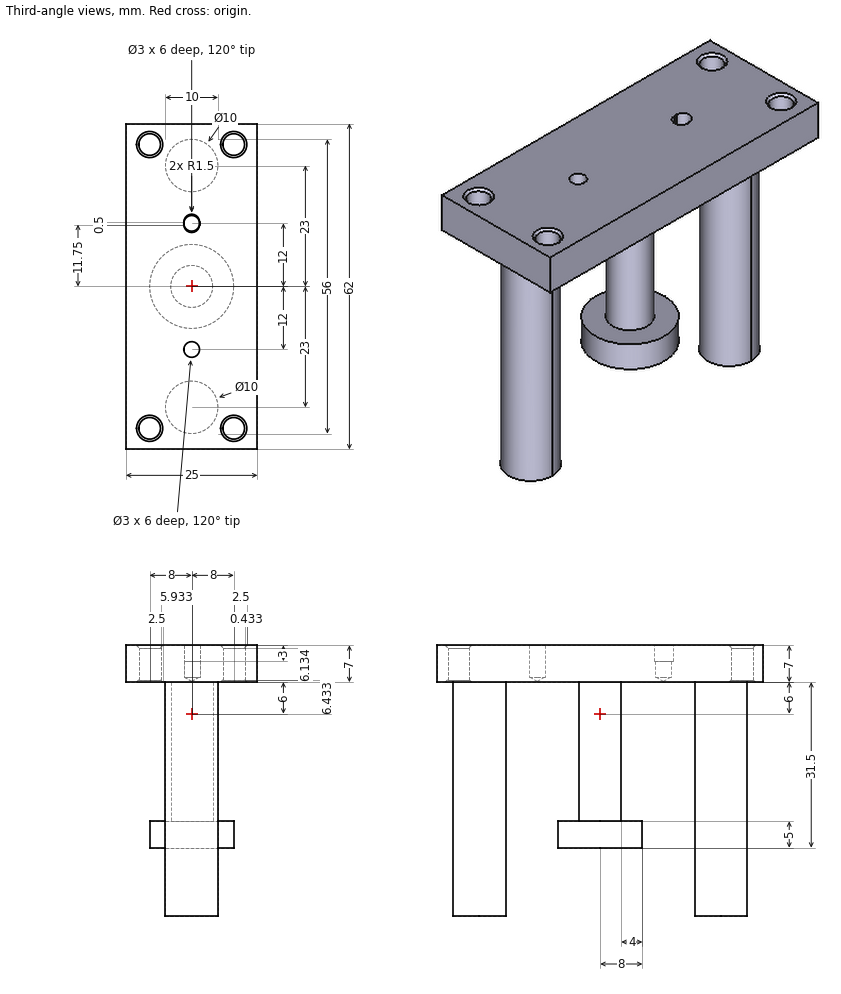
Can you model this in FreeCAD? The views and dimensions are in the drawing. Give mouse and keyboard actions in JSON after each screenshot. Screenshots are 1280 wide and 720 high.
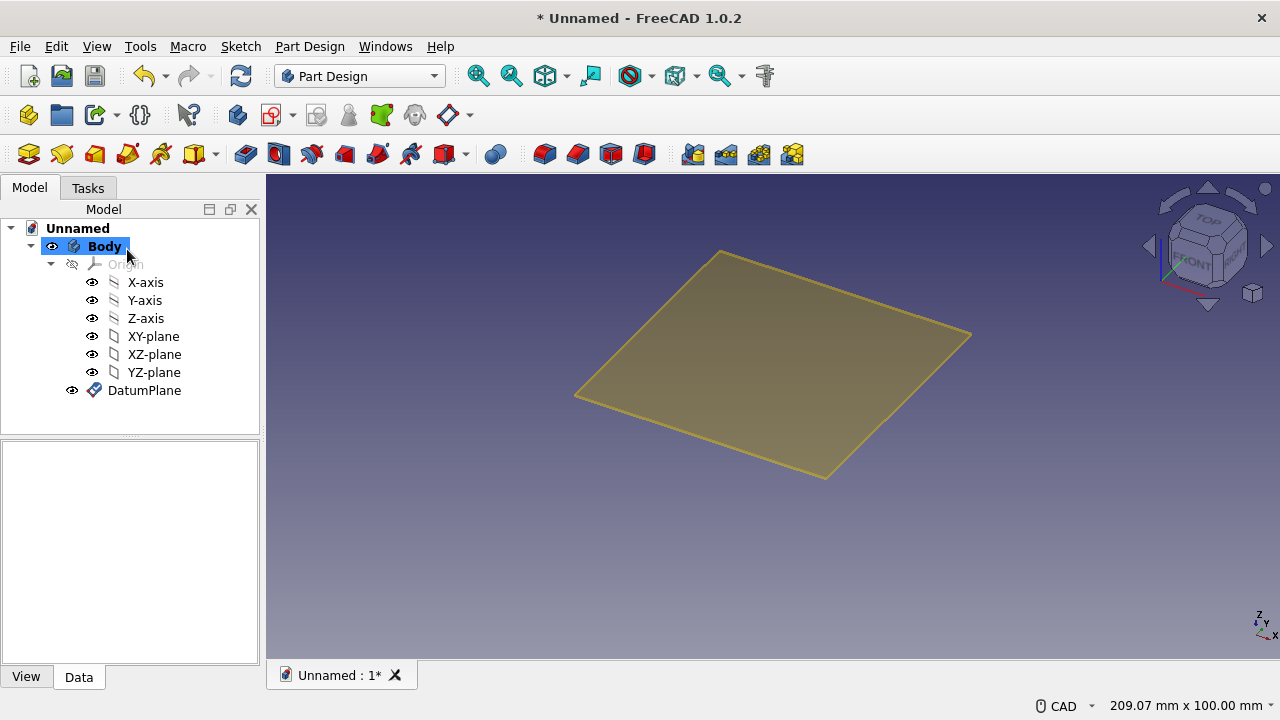
{"action": "left_click", "coordinate": [117, 390]}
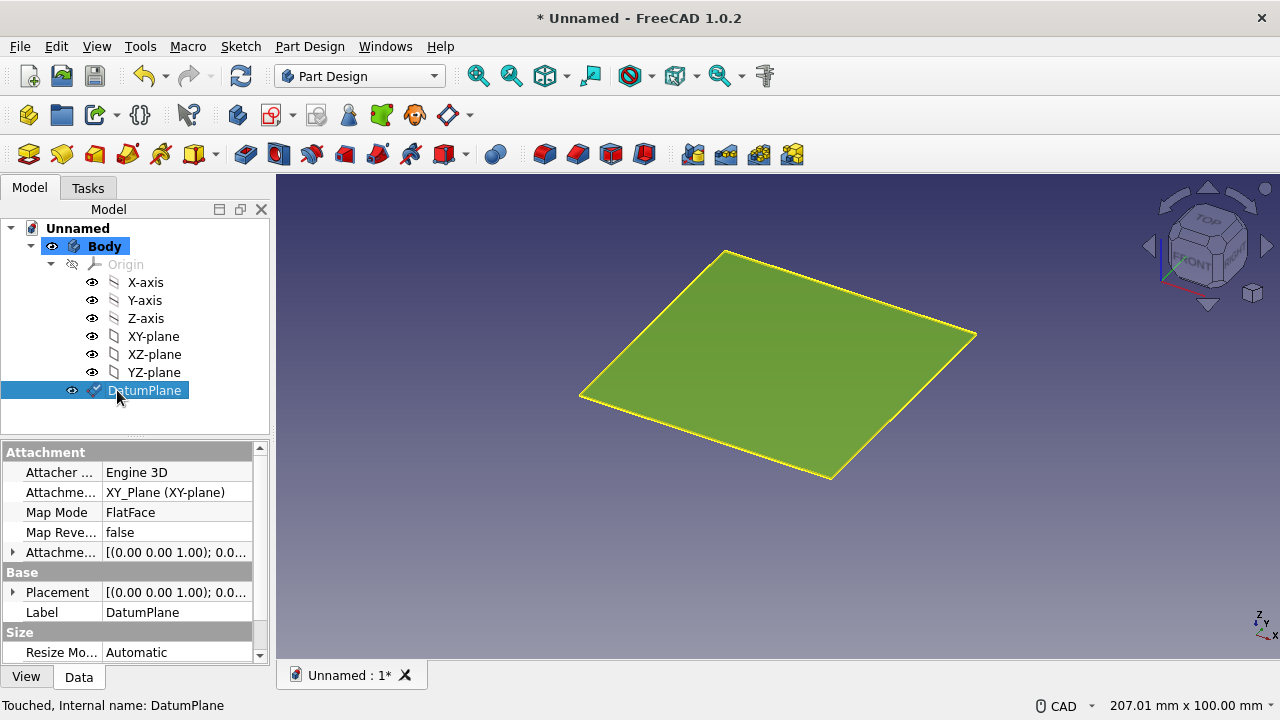
{"action": "left_click", "coordinate": [270, 116]}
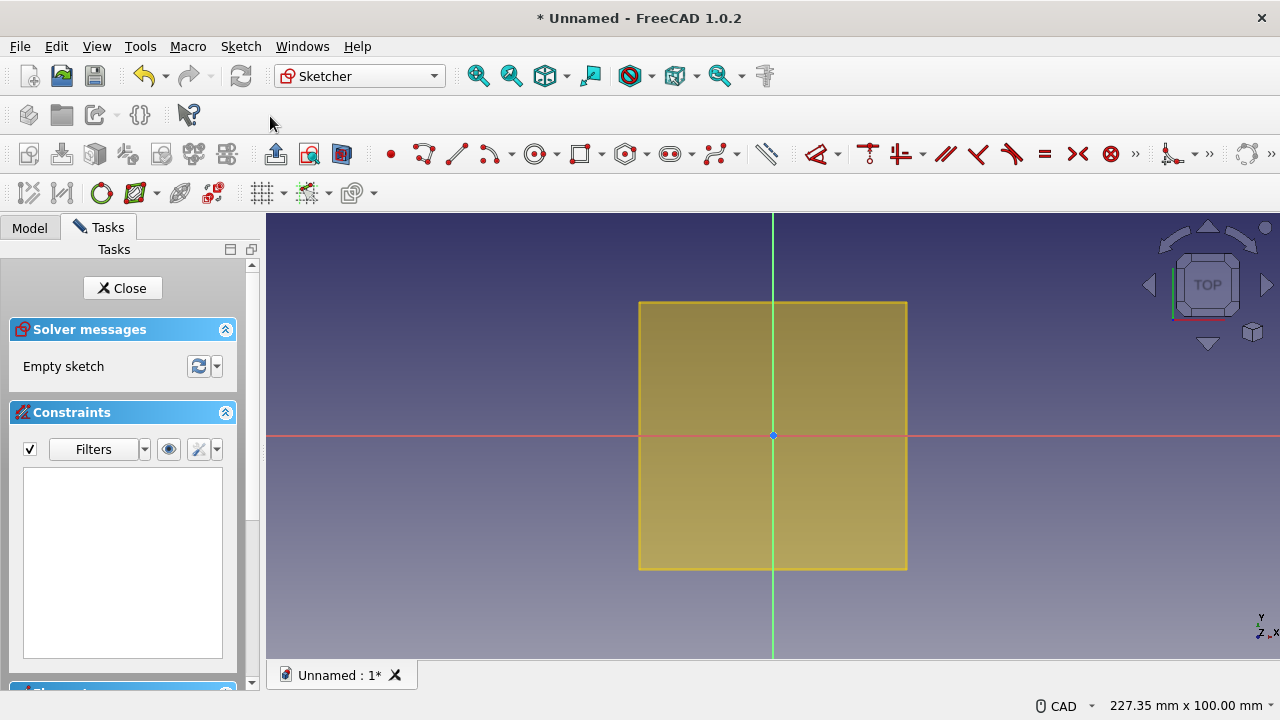
{"action": "left_click", "coordinate": [602, 154]}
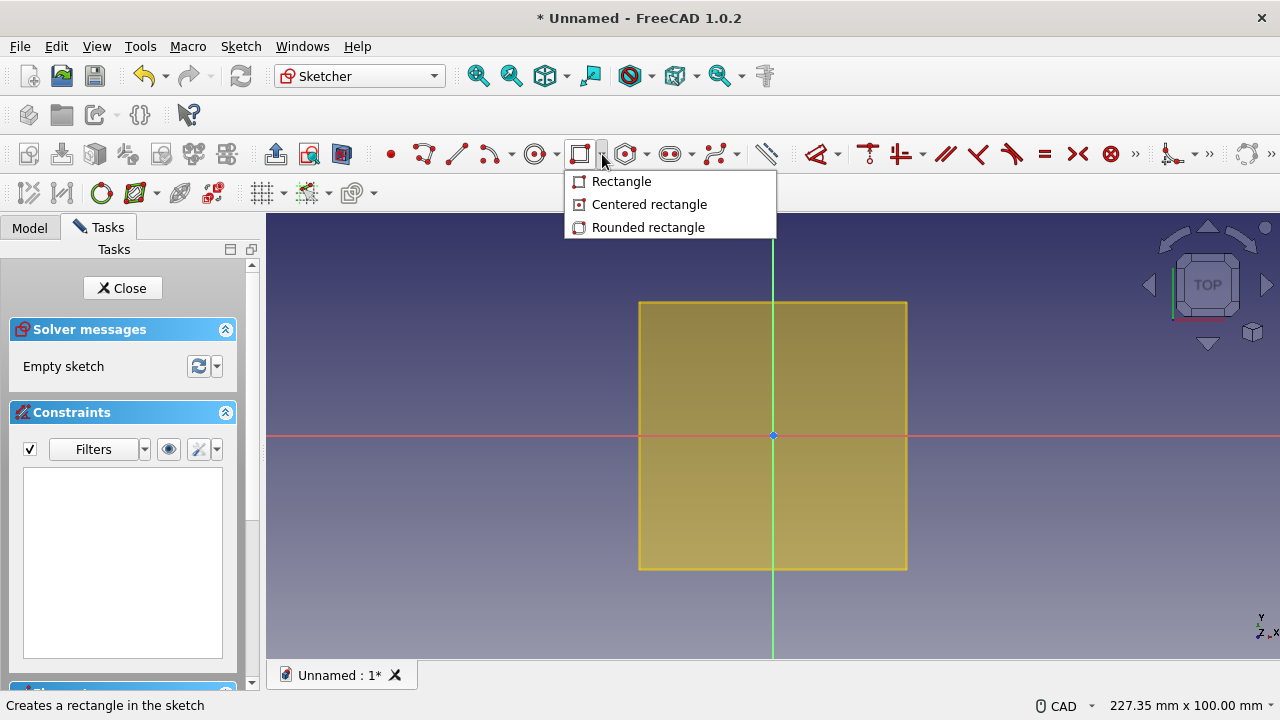
{"action": "left_click", "coordinate": [670, 204]}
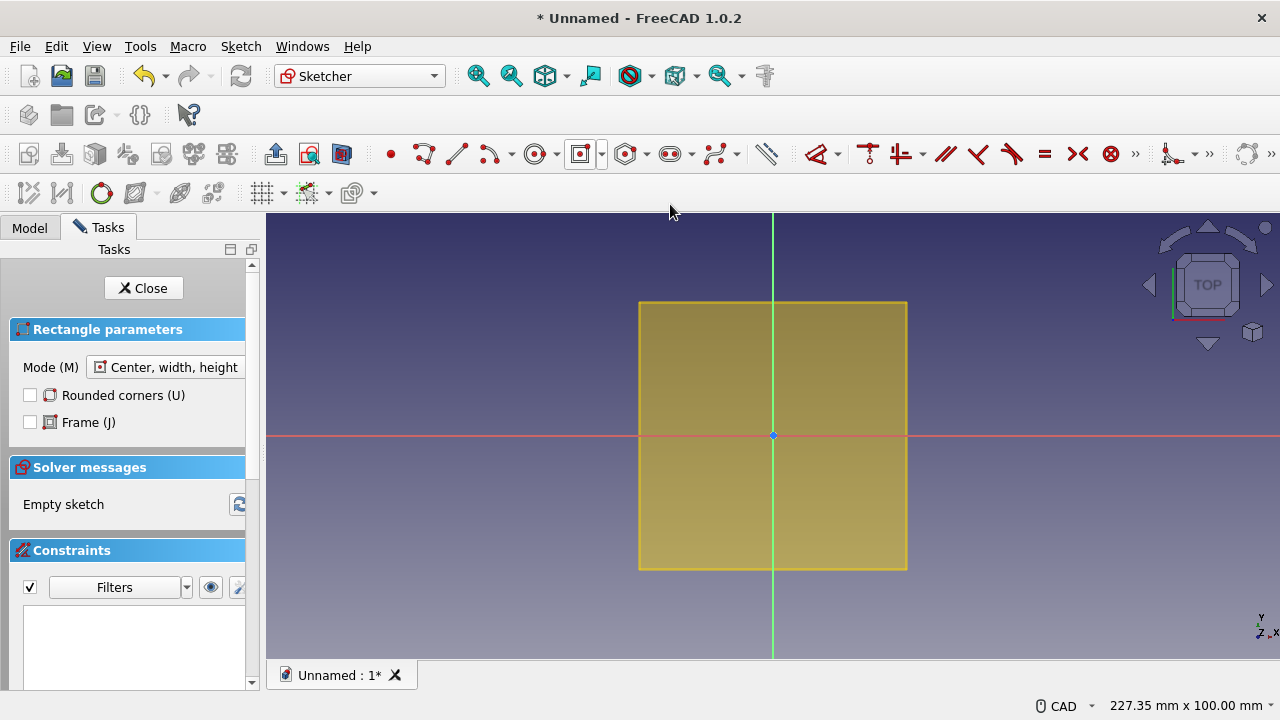
{"action": "left_click", "coordinate": [773, 436]}
{"action": "left_click", "coordinate": [829, 298]}
{"action": "key", "text": "Escape"}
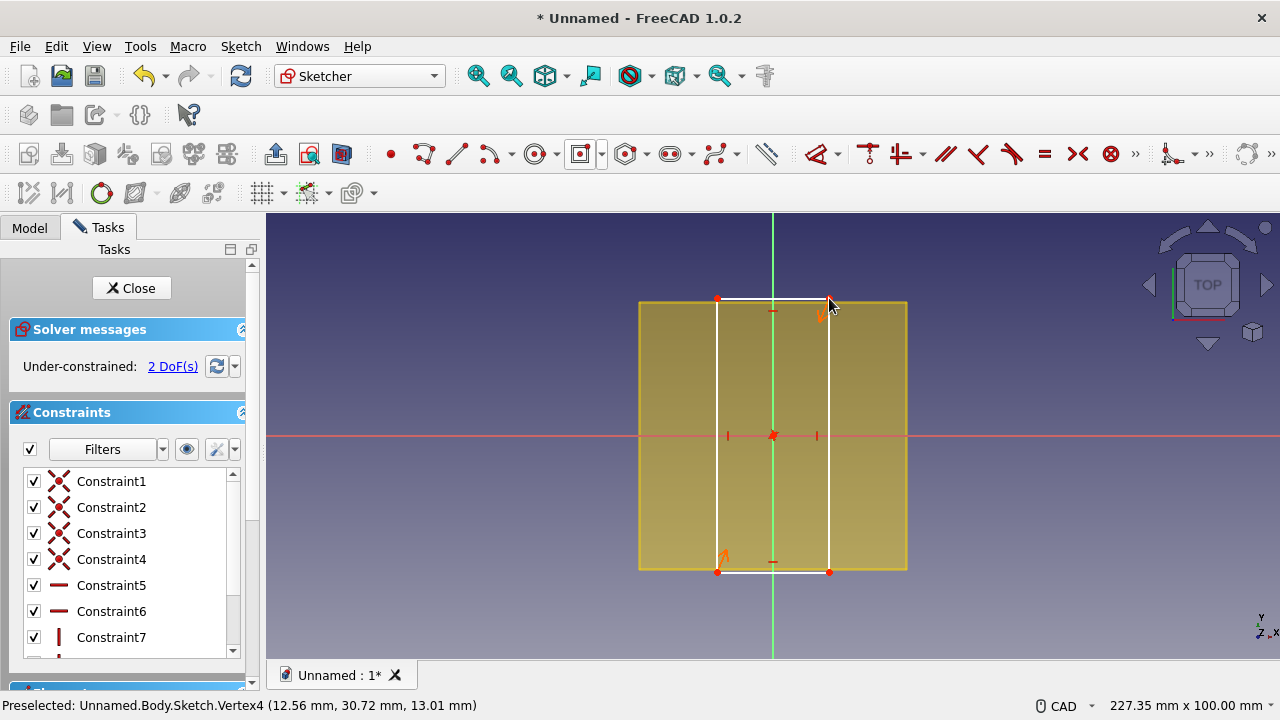
{"action": "left_click", "coordinate": [816, 154]}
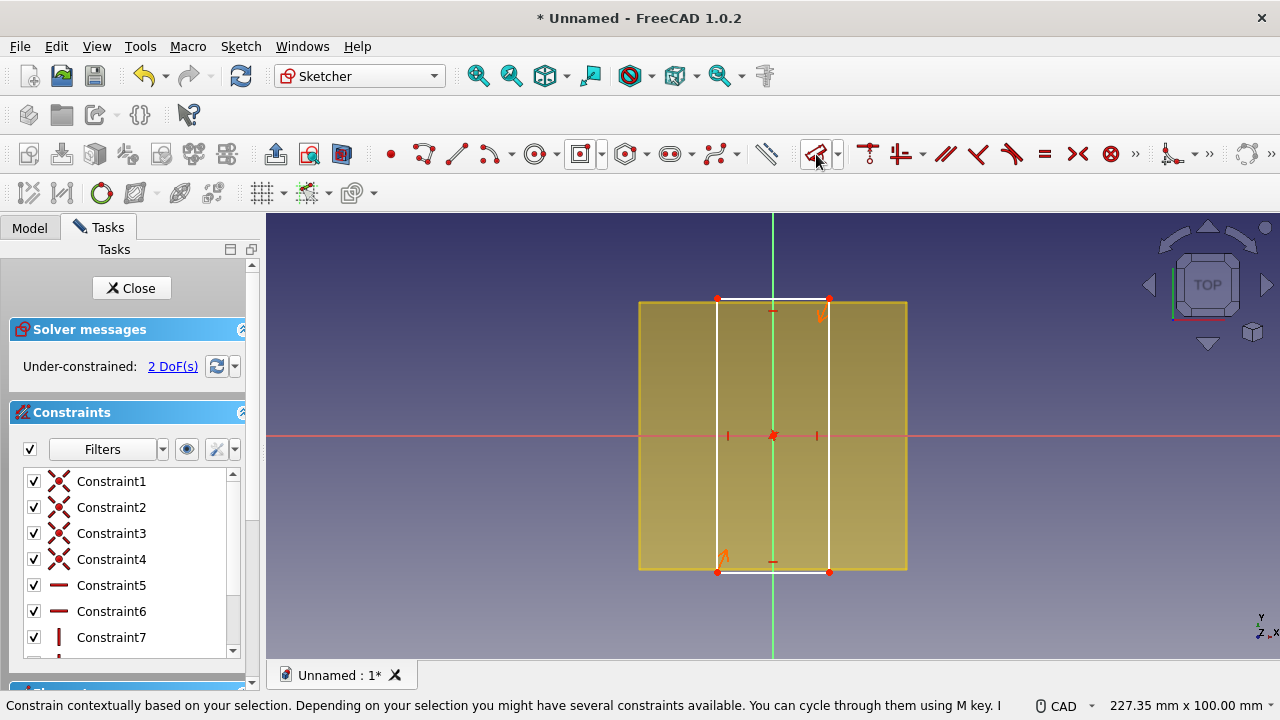
{"action": "left_click", "coordinate": [751, 573]}
{"action": "left_click", "coordinate": [747, 607]}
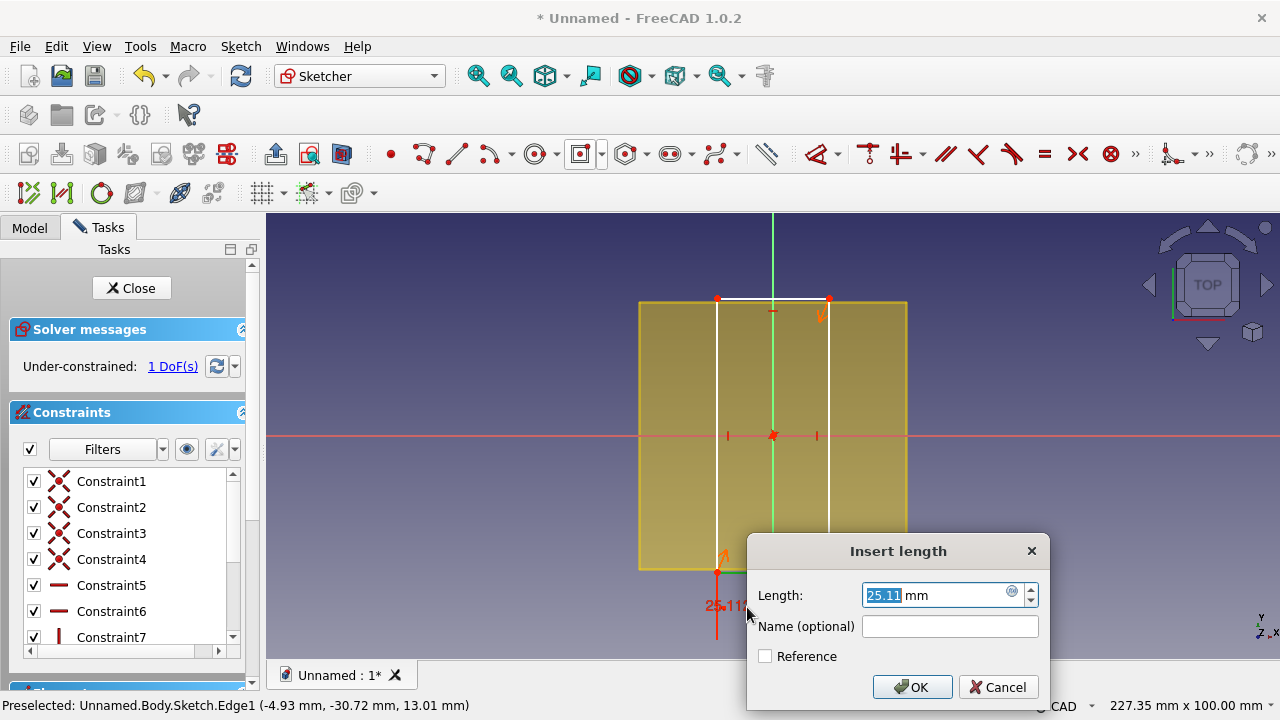
{"action": "type", "text": "25"}
{"action": "key", "text": "Return"}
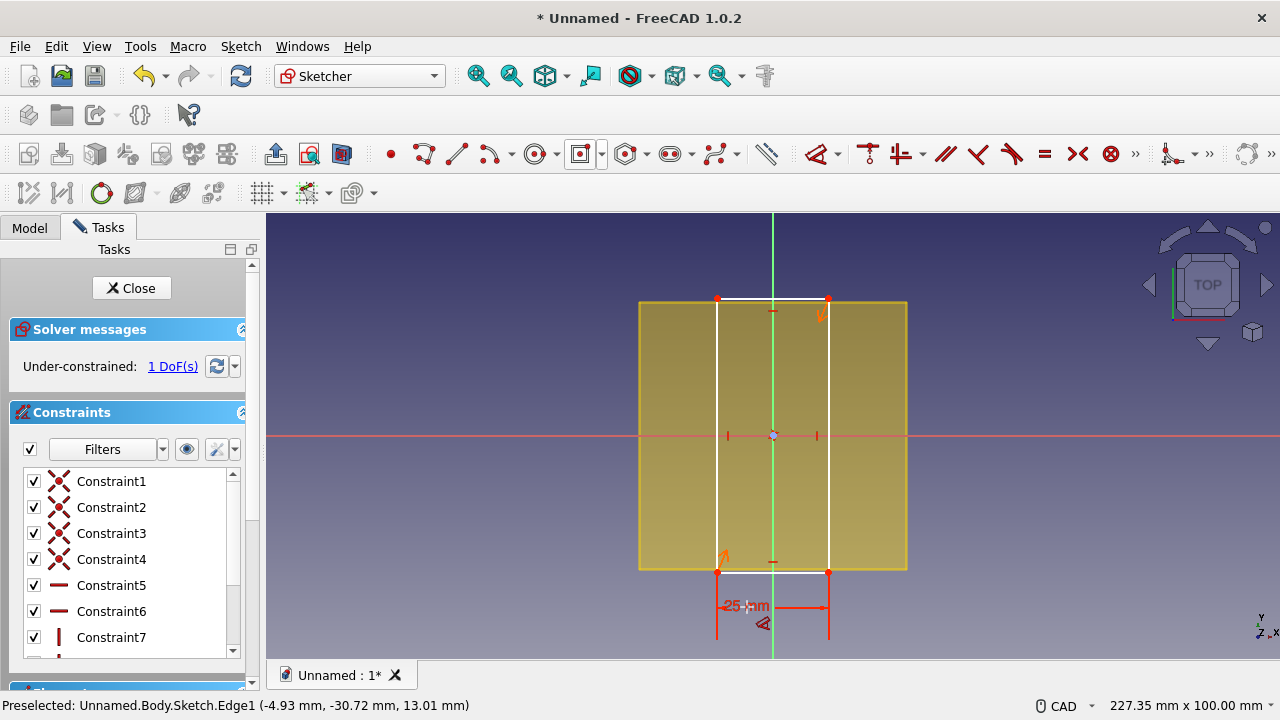
{"action": "left_click", "coordinate": [829, 491]}
{"action": "left_click", "coordinate": [863, 373]}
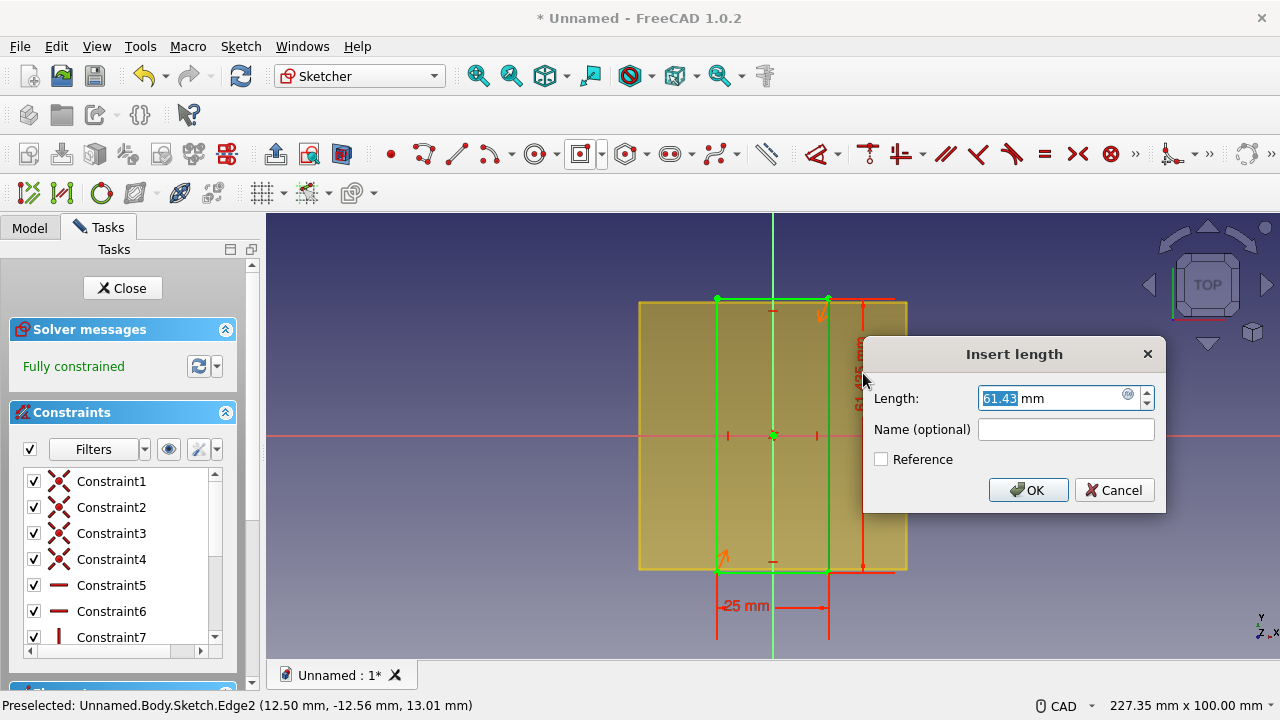
{"action": "type", "text": "62"}
{"action": "key", "text": "Return"}
{"action": "key", "text": "Escape"}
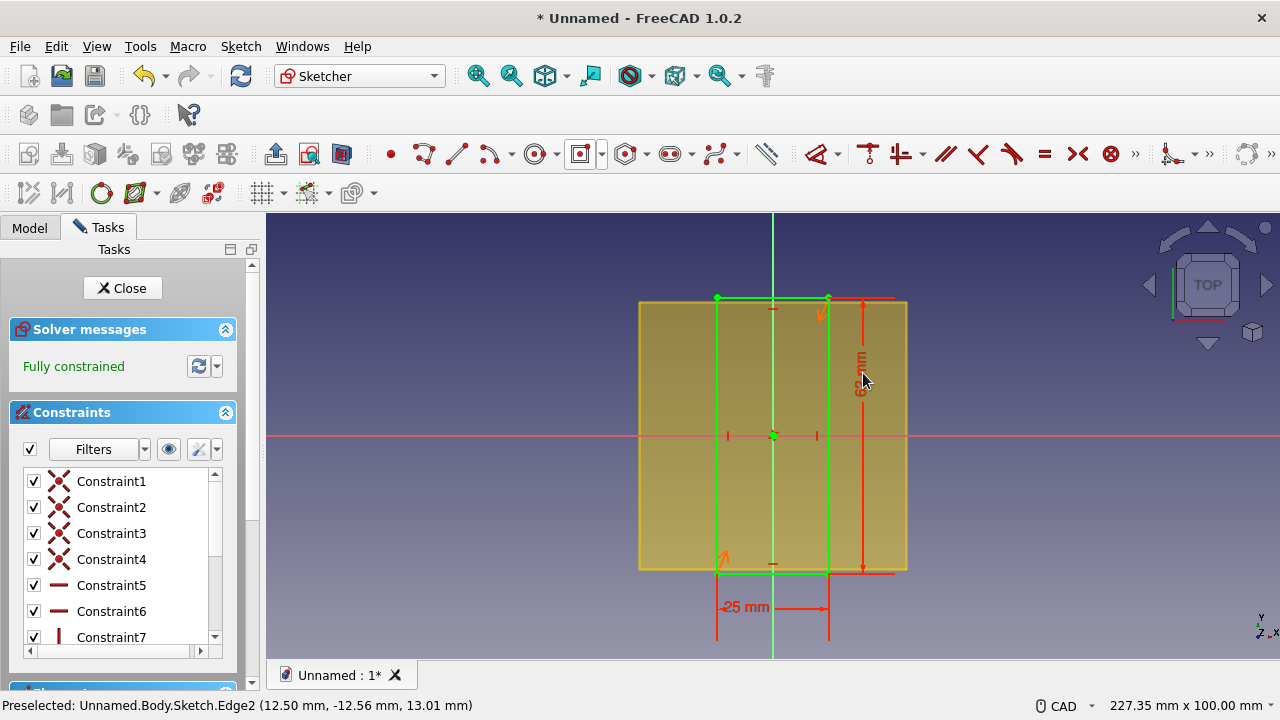
{"action": "left_click", "coordinate": [123, 288]}